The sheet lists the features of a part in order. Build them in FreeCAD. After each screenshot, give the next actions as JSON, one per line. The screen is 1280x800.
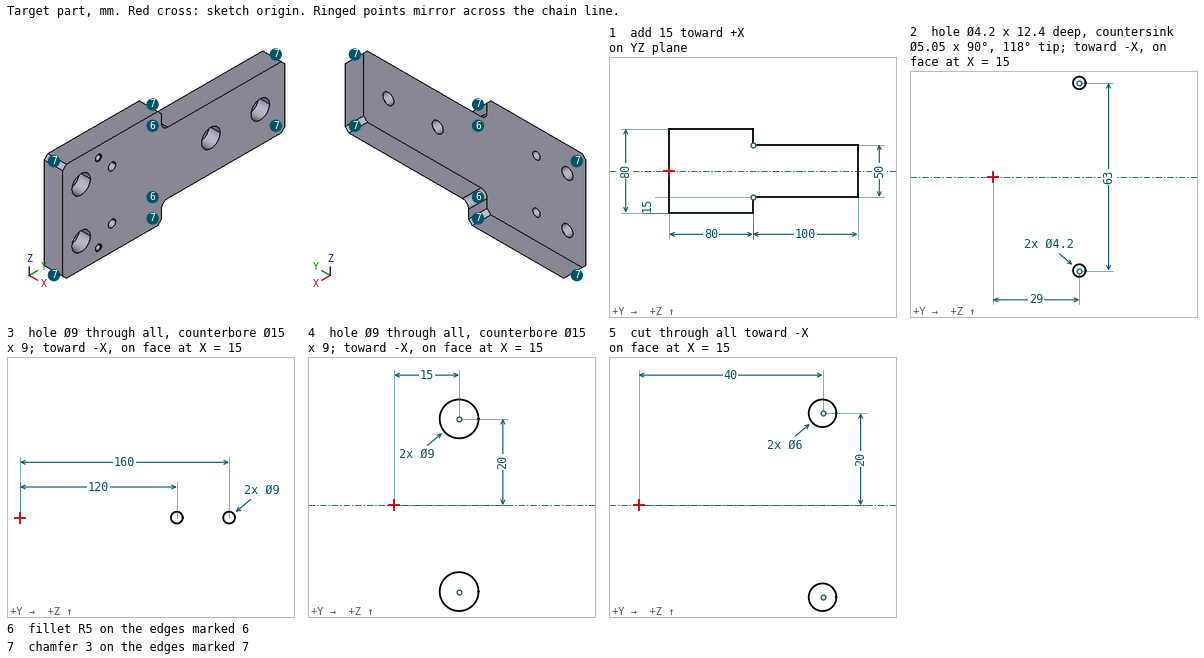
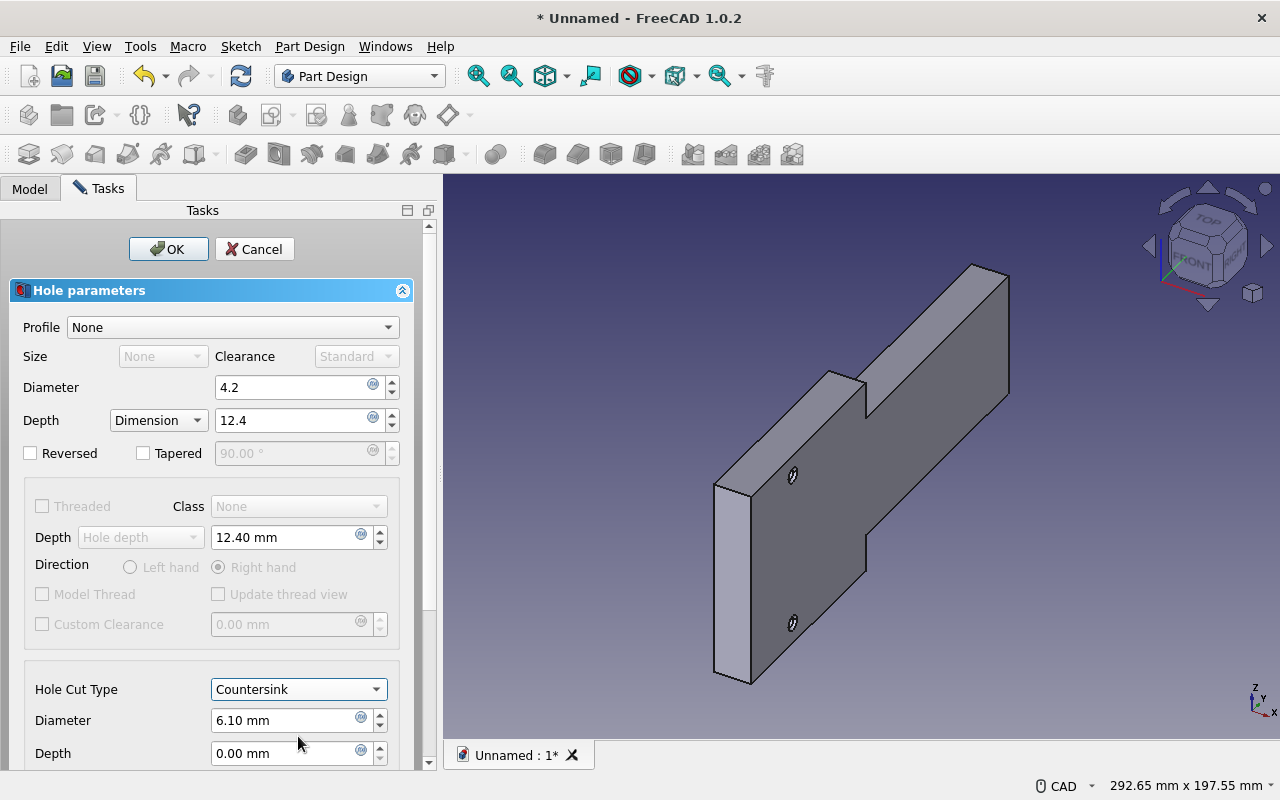
{"action": "triple_click", "coordinate": [292, 720]}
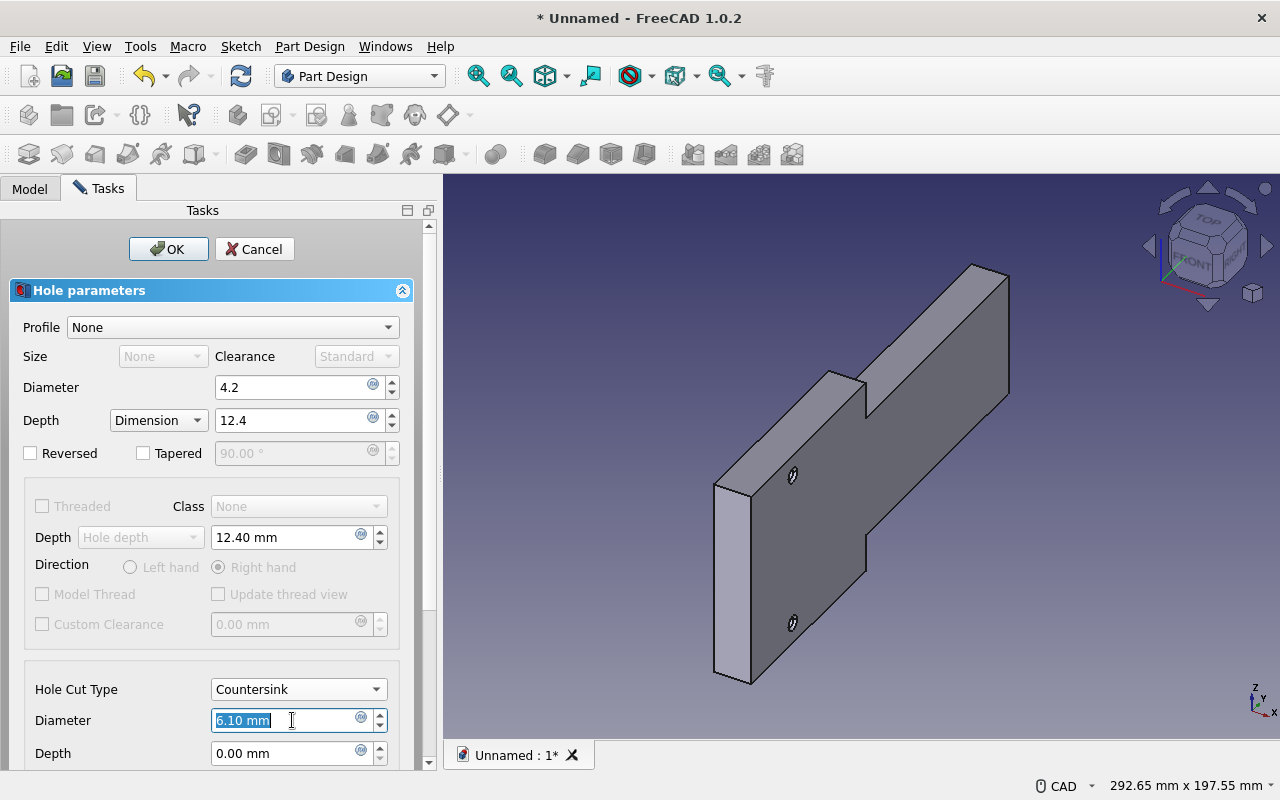
{"action": "type", "text": "5.05"}
{"action": "key", "text": "Tab"}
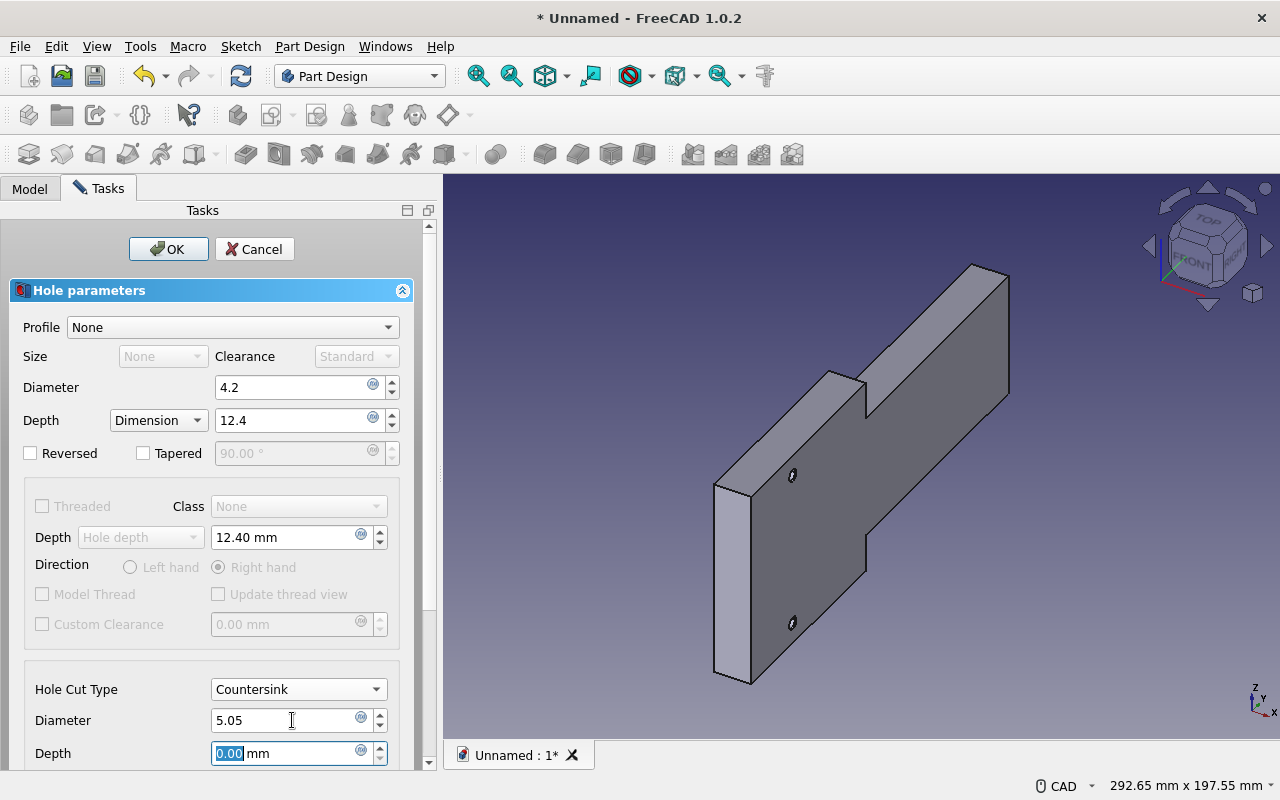
{"action": "left_click", "coordinate": [169, 249]}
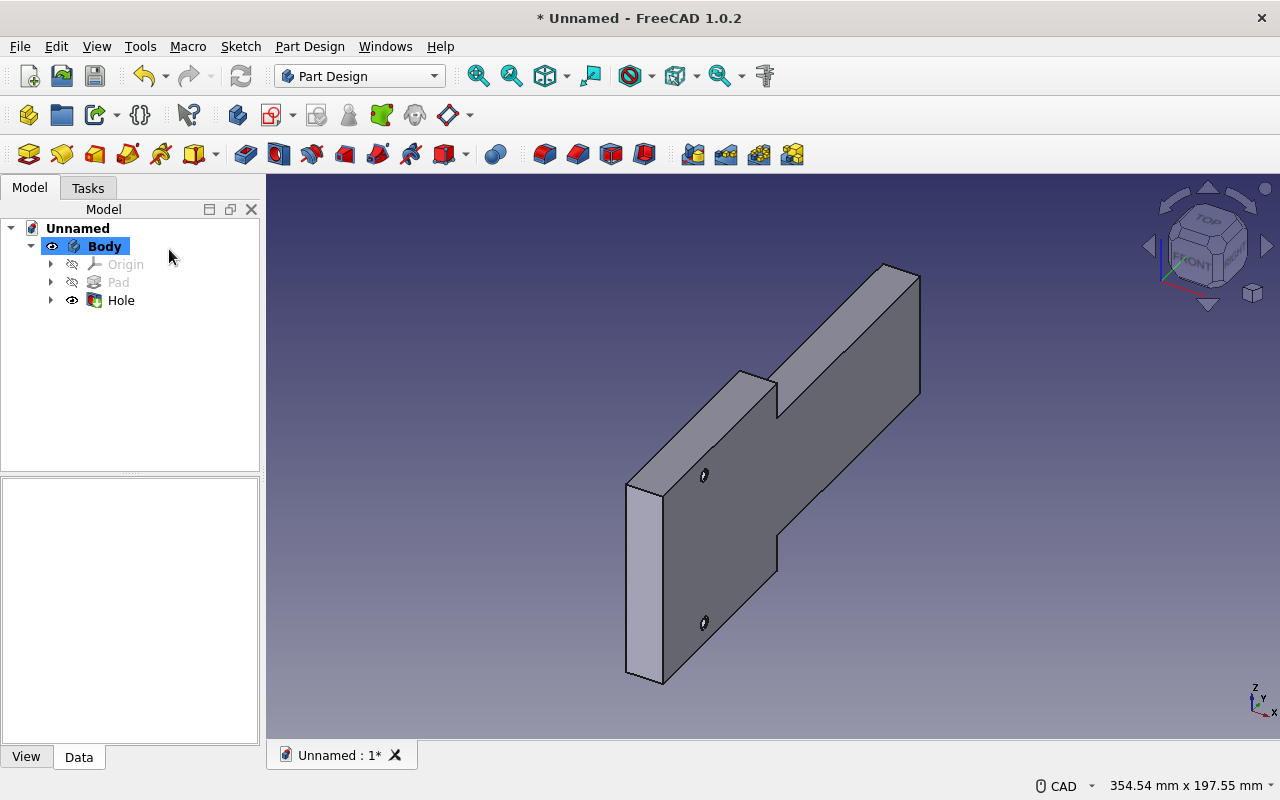
{"action": "left_click", "coordinate": [718, 535]}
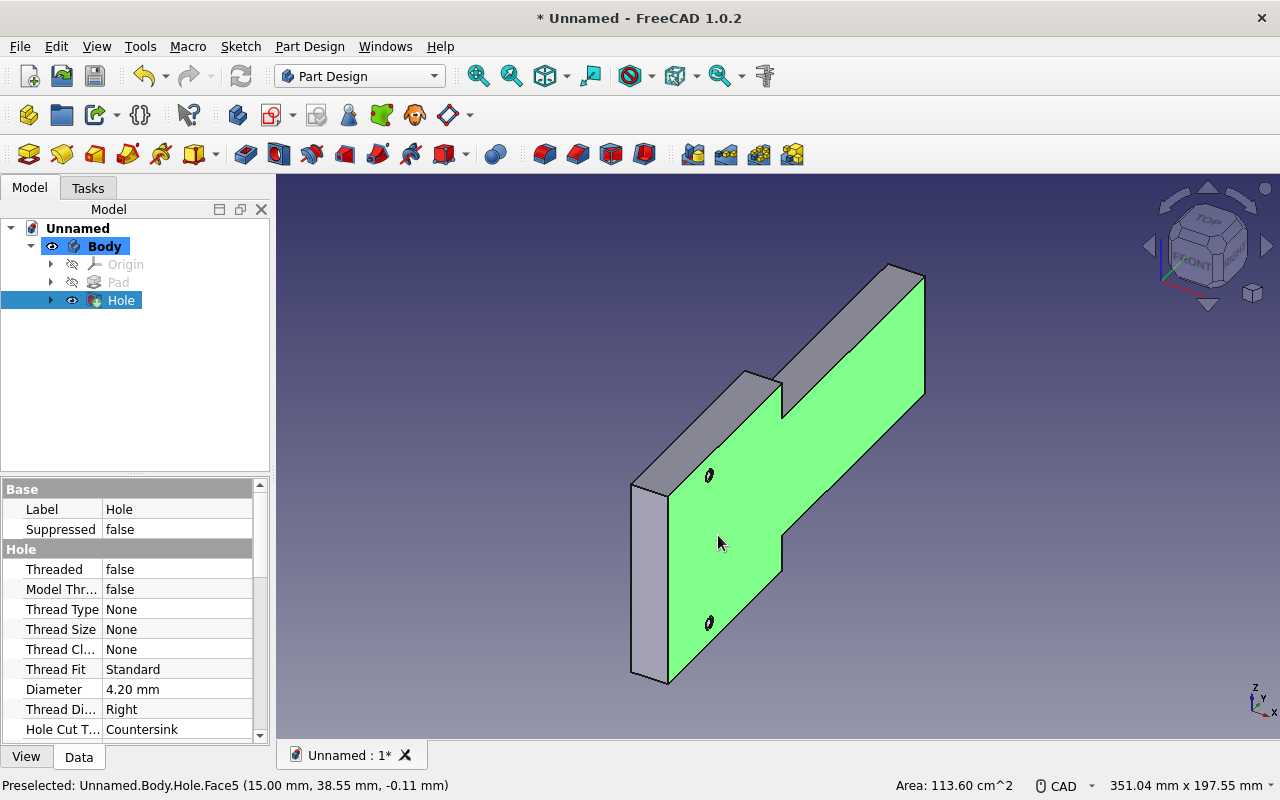
{"action": "left_click", "coordinate": [270, 116]}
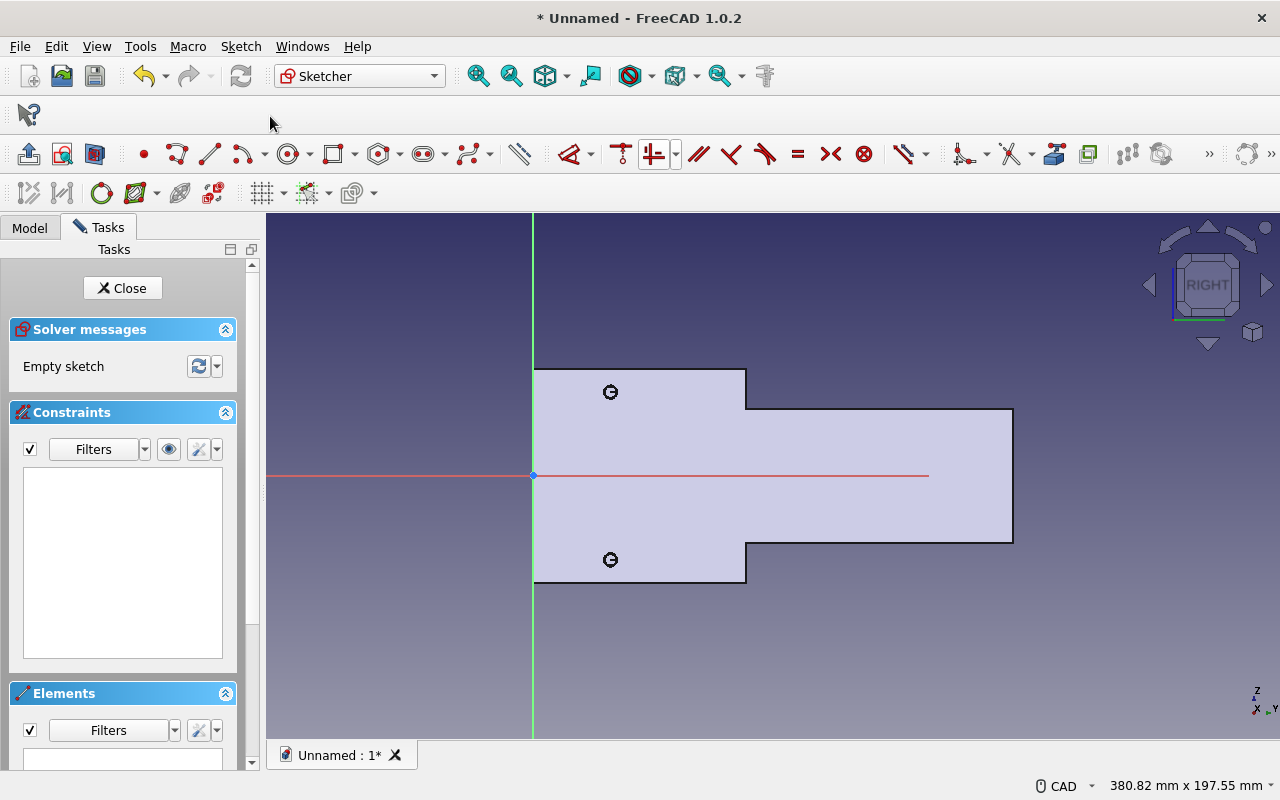
{"action": "scroll", "coordinate": [972, 476], "scroll_direction": "up", "scroll_amount": 7}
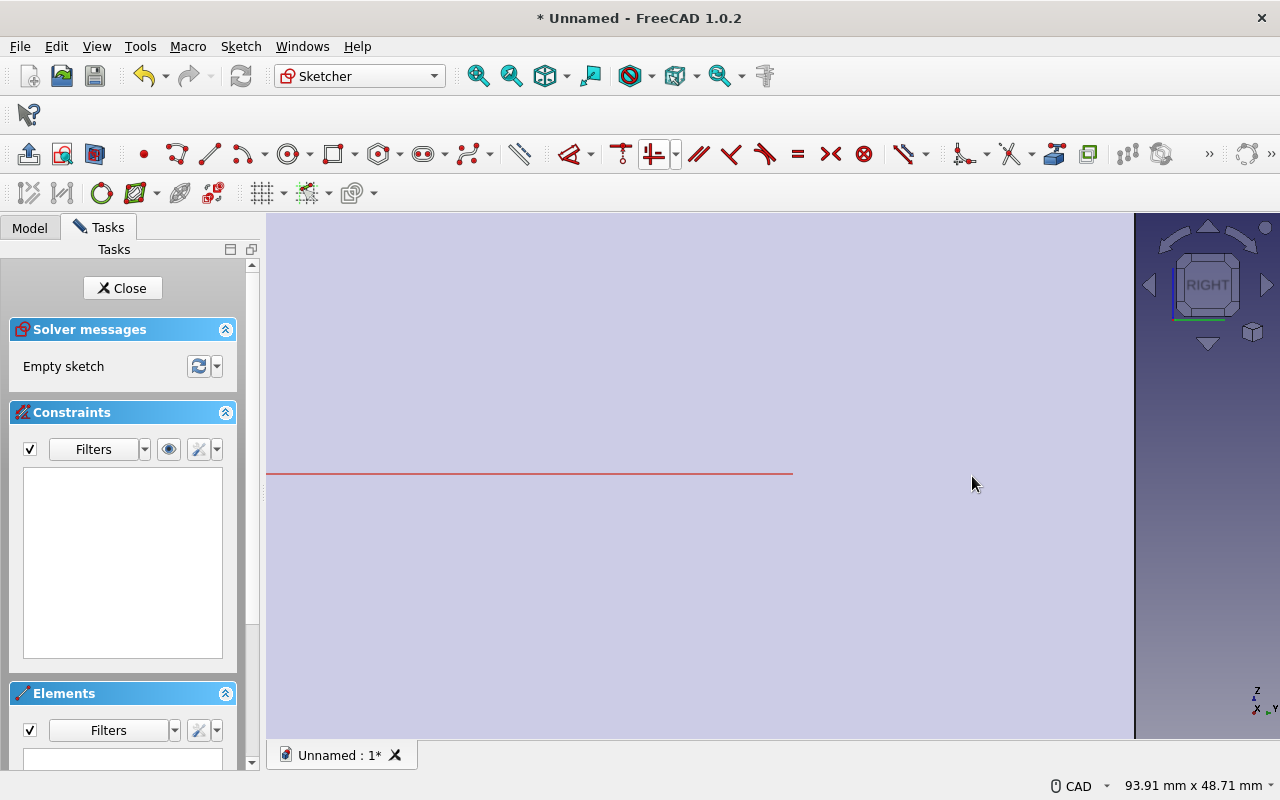
{"action": "key", "text": "g c"}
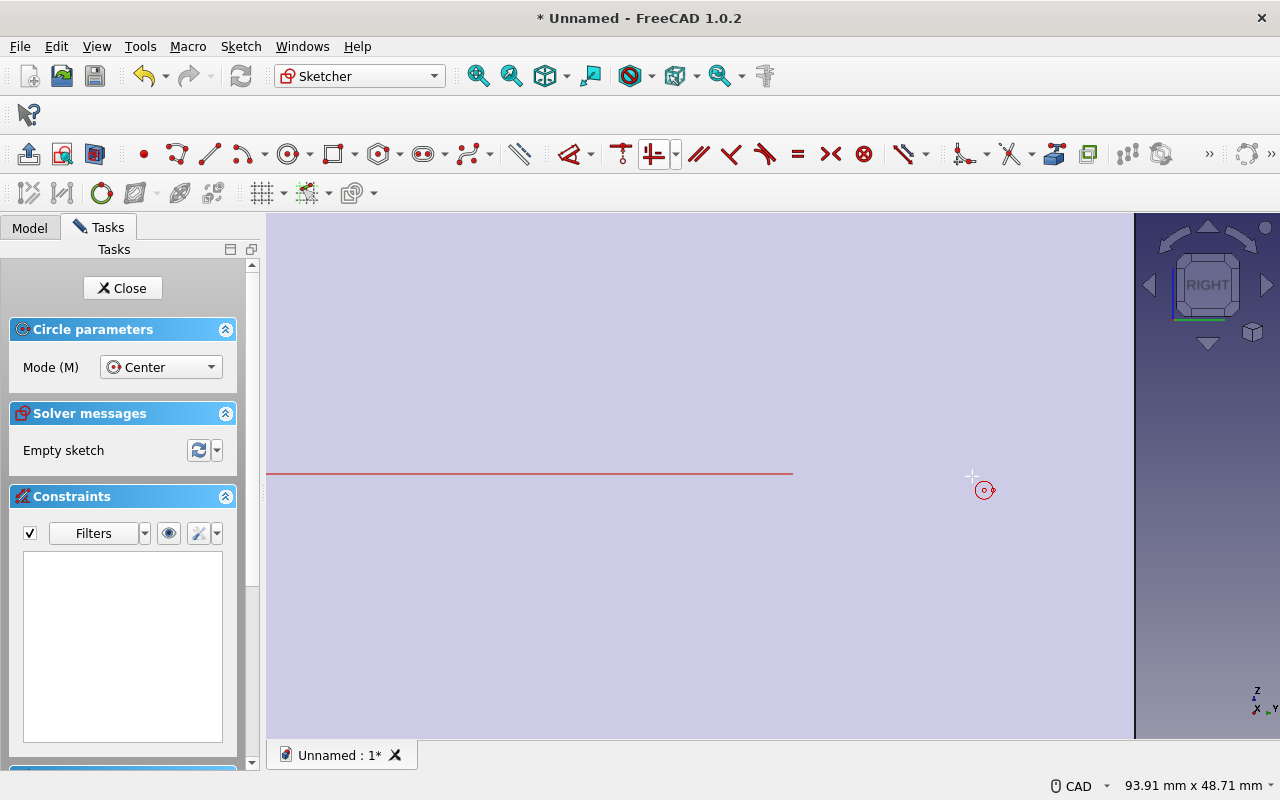
{"action": "left_click", "coordinate": [919, 474]}
{"action": "mouse_move", "coordinate": [953, 440]}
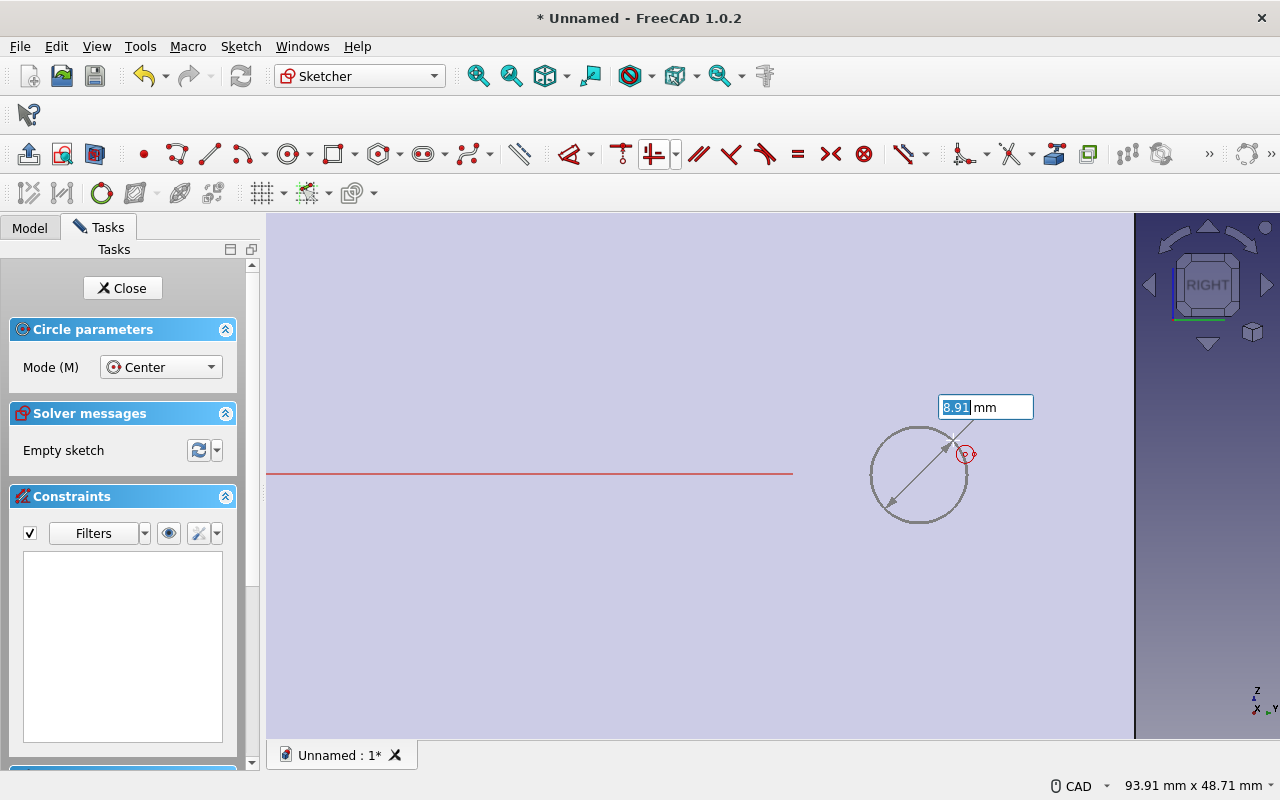
{"action": "type", "text": "9"}
{"action": "key", "text": "Return"}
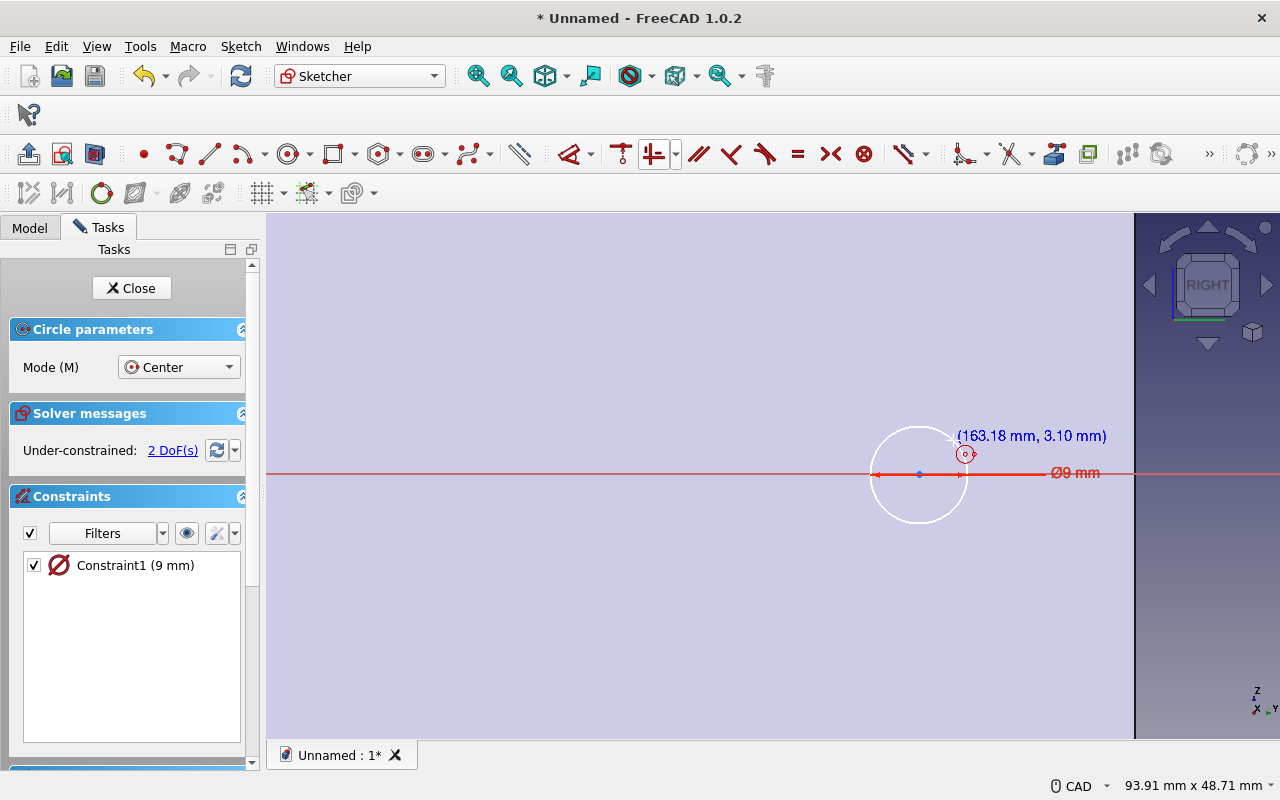
{"action": "left_click", "coordinate": [487, 474]}
{"action": "mouse_move", "coordinate": [521, 440]}